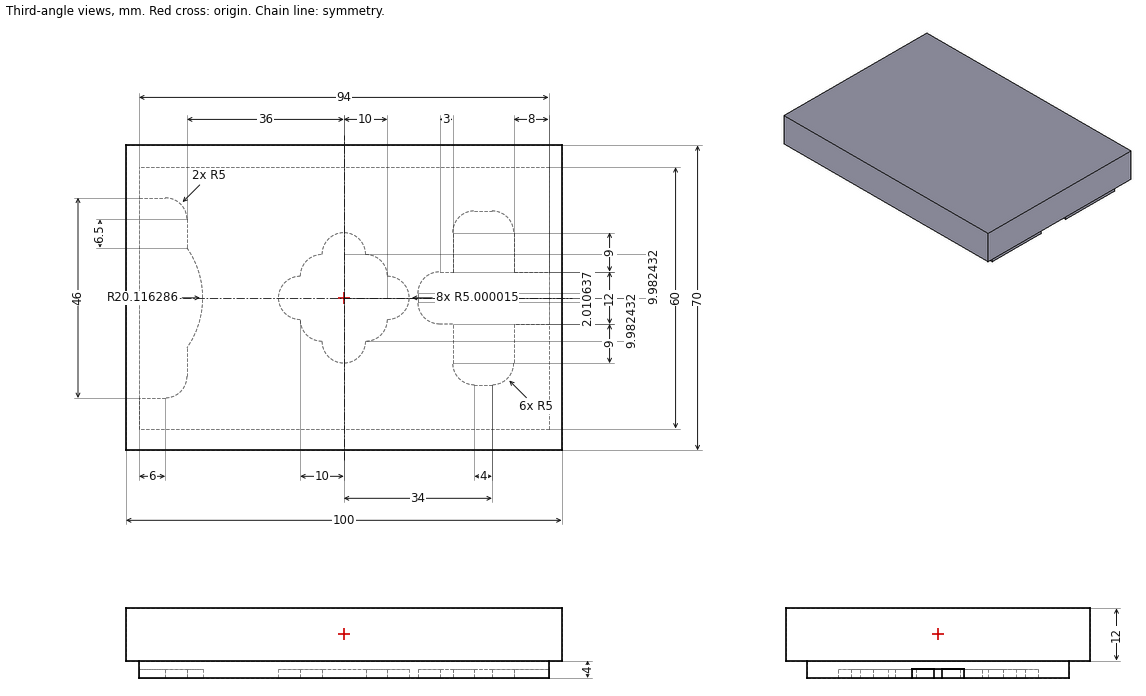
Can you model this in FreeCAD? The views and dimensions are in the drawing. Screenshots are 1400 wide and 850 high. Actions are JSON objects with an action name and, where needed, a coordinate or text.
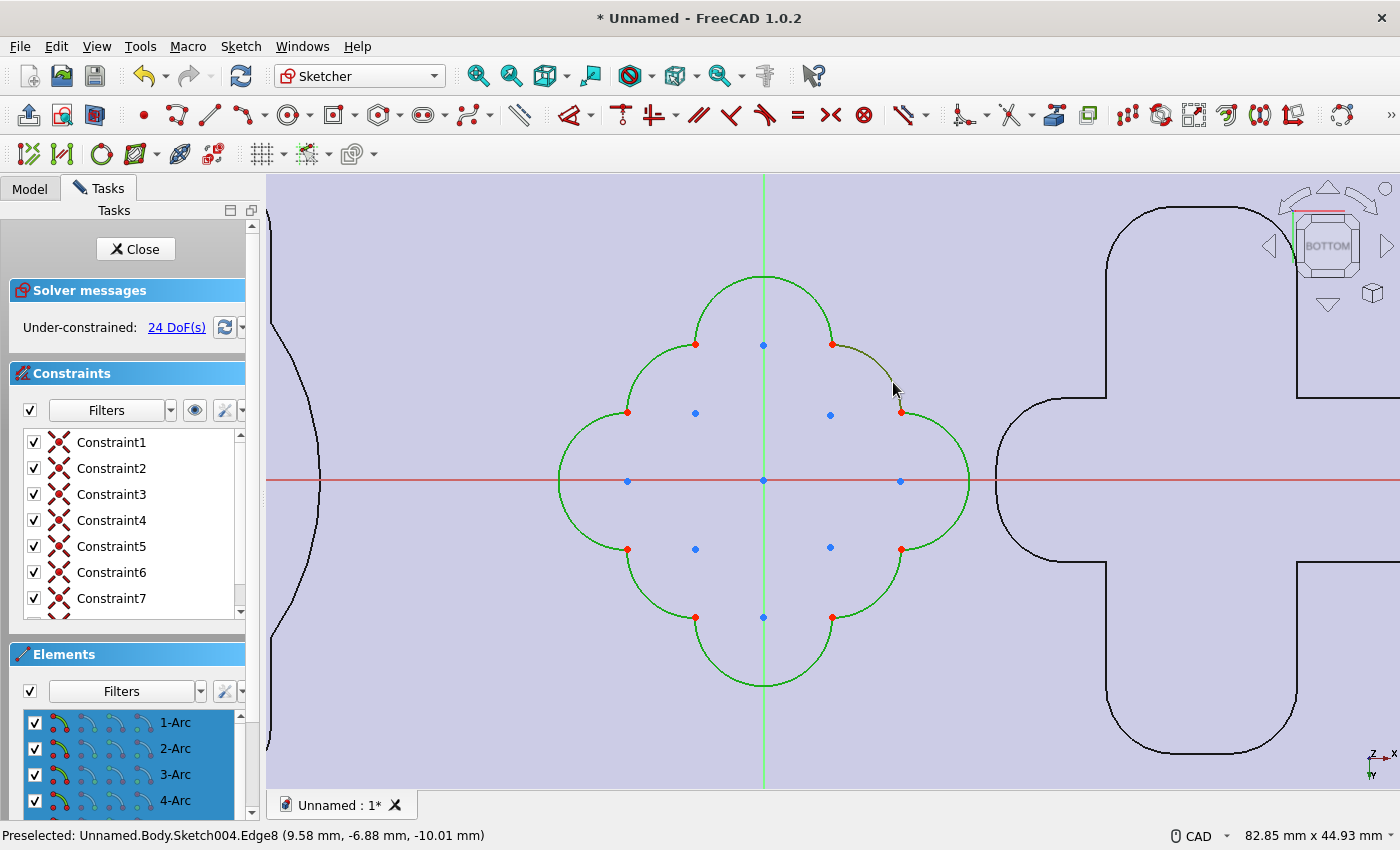
{"action": "left_click", "coordinate": [798, 116]}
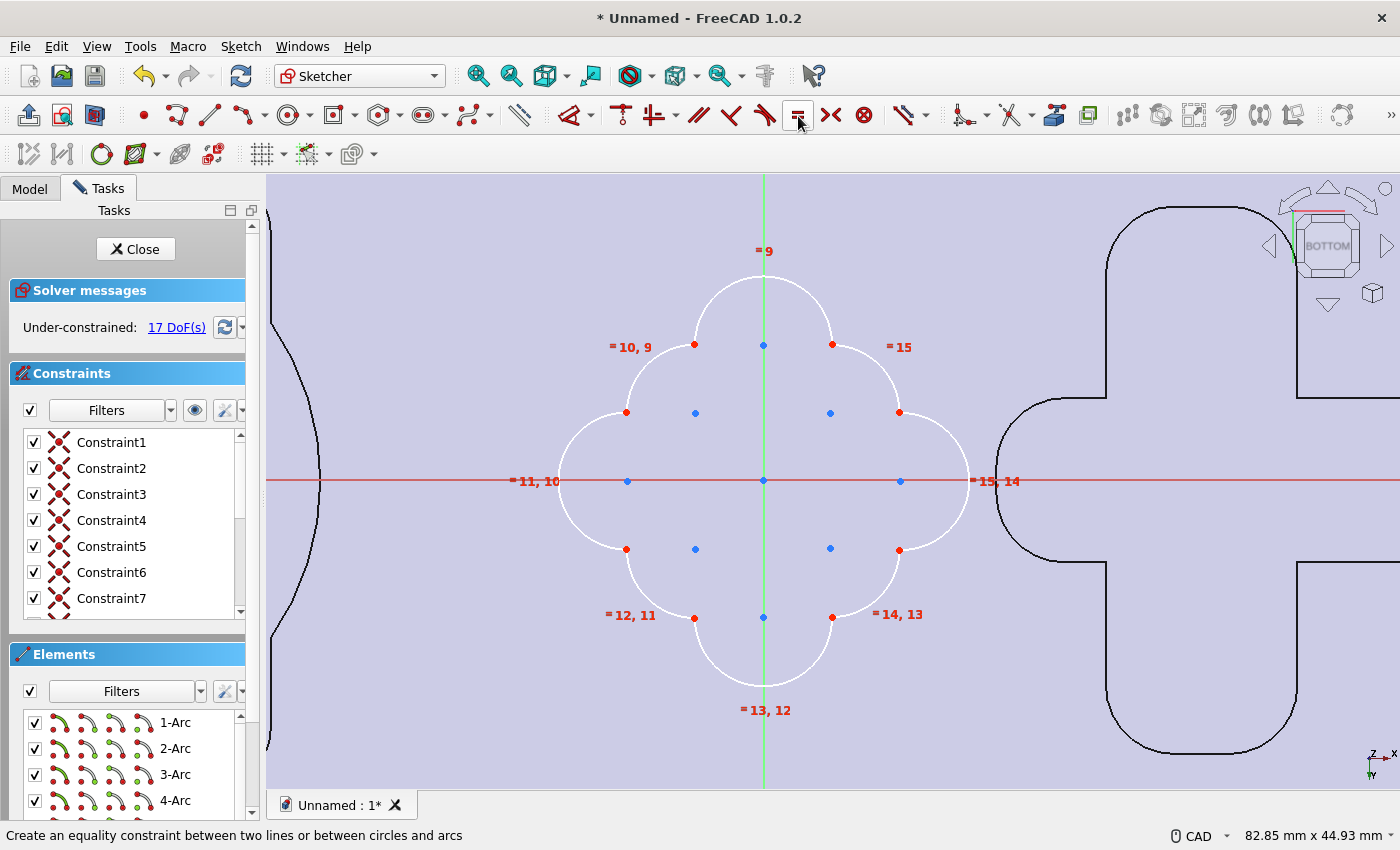
{"action": "left_click", "coordinate": [764, 345]}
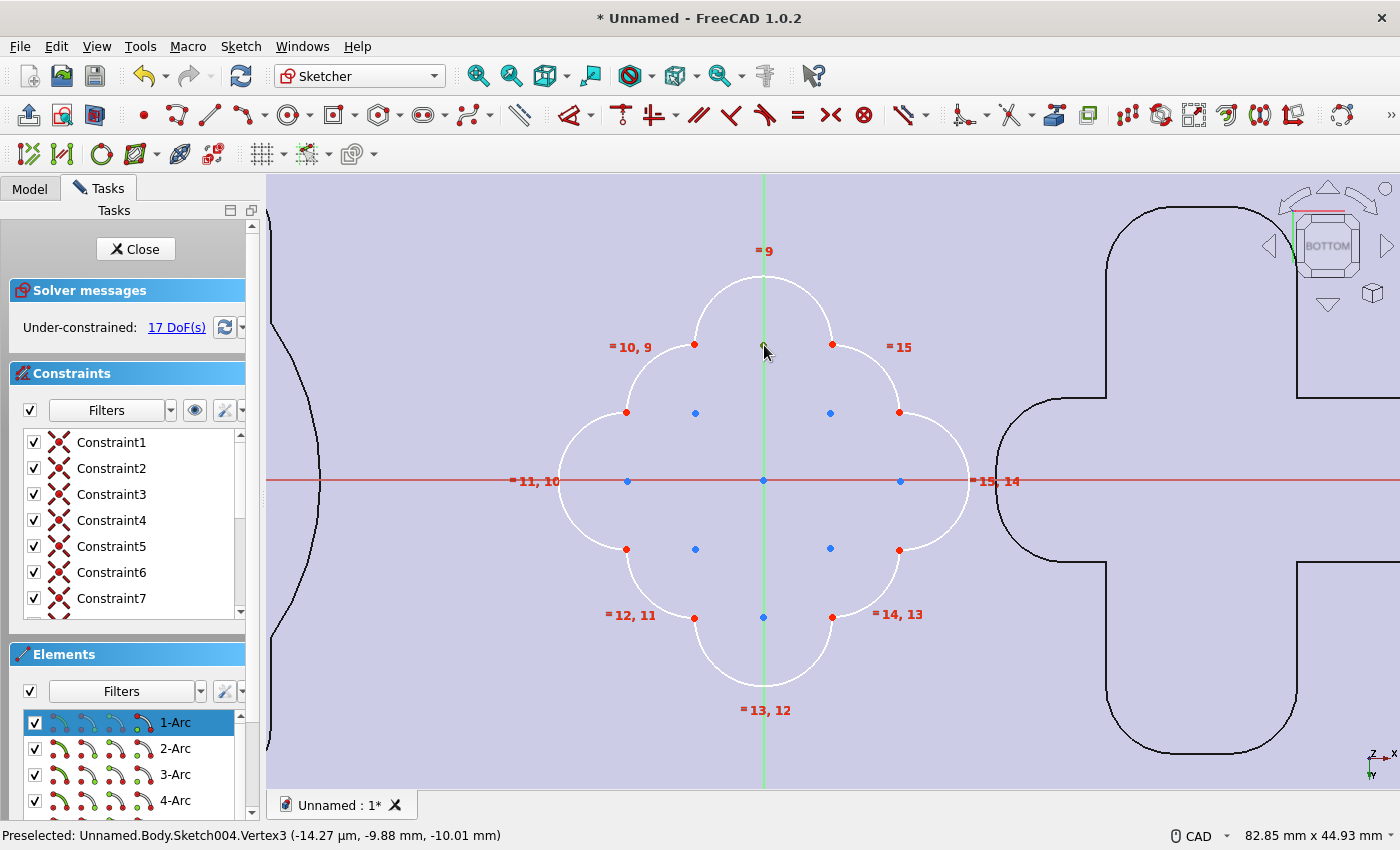
{"action": "left_click", "coordinate": [764, 721]}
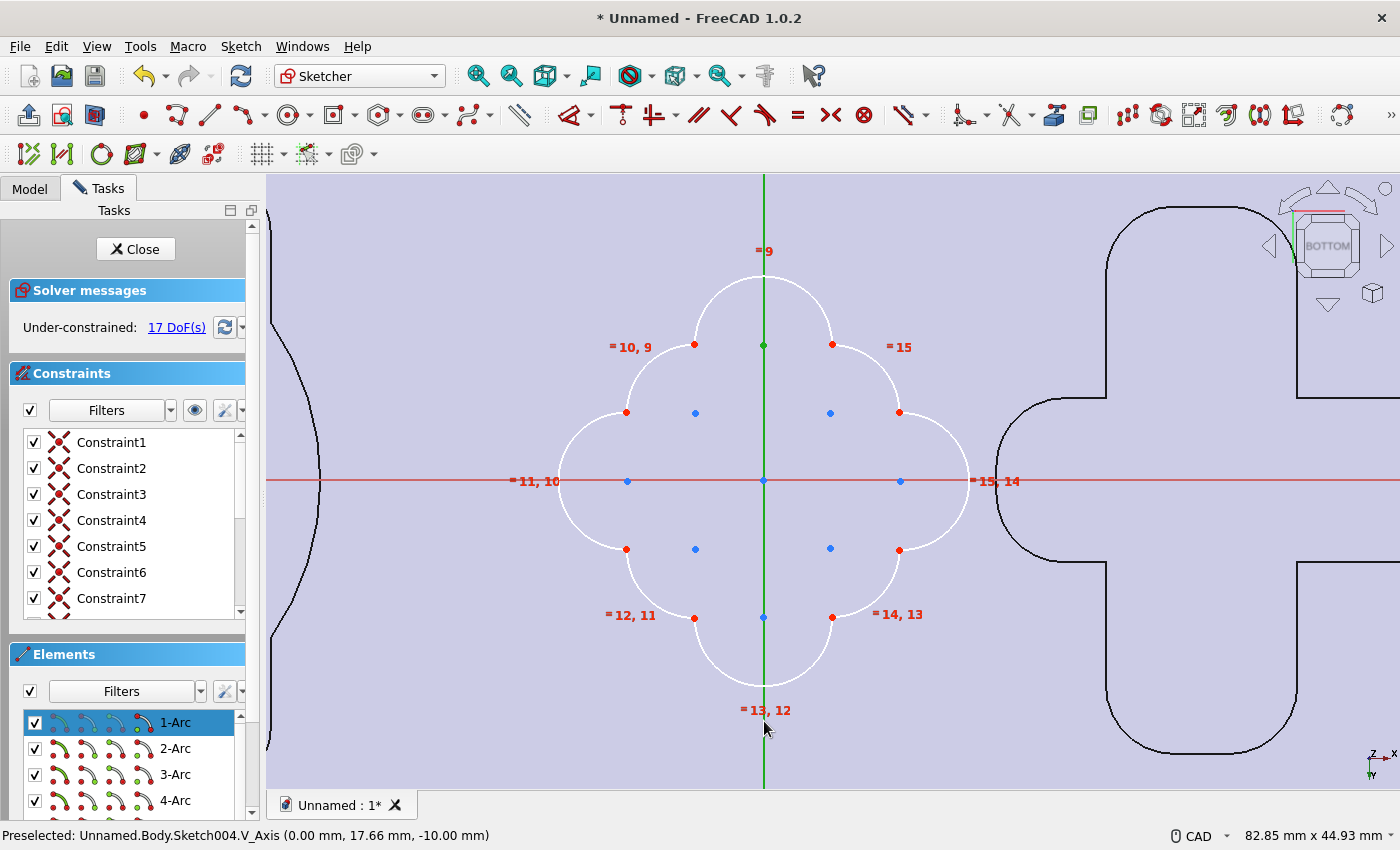
{"action": "left_click", "coordinate": [621, 116]}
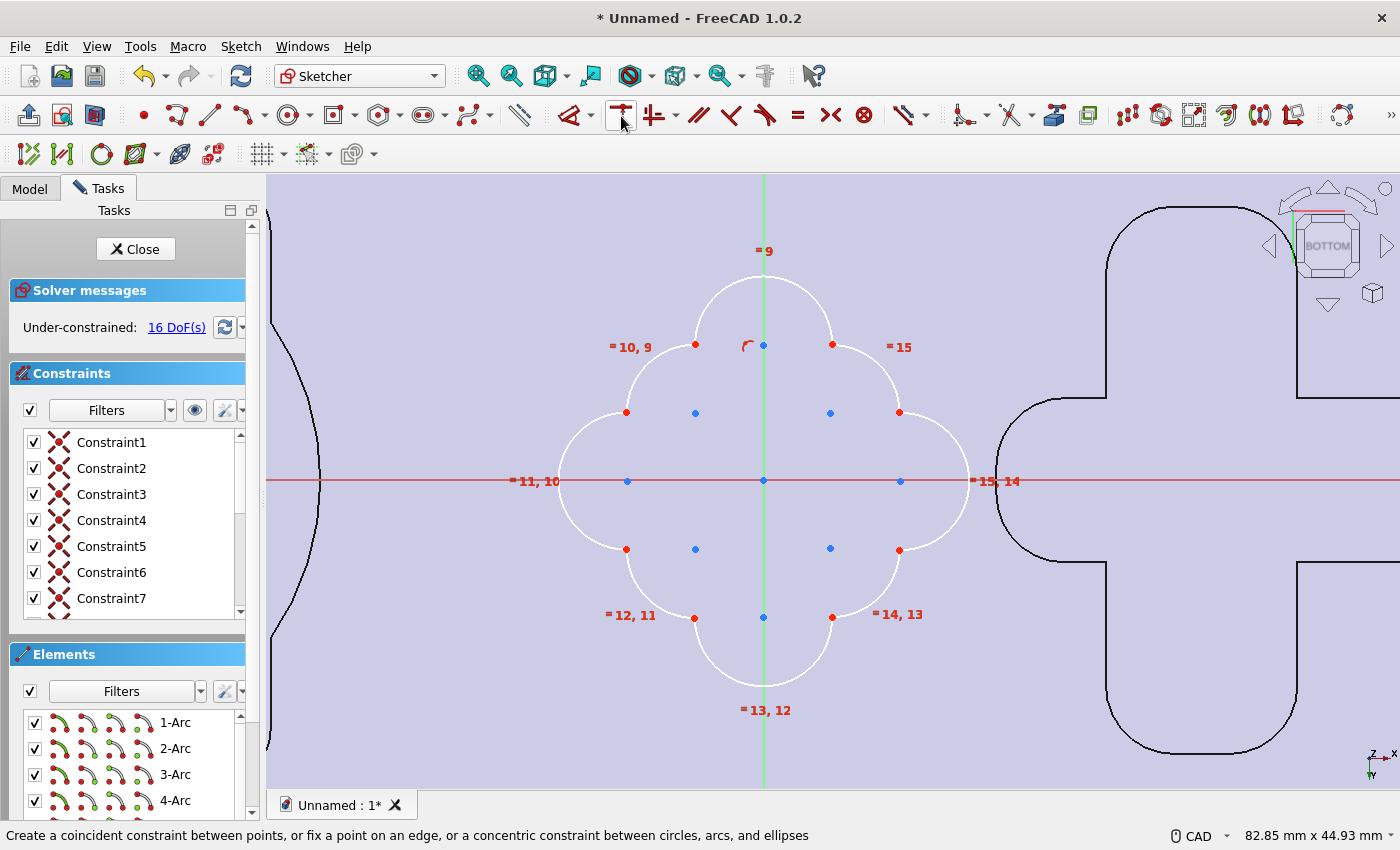
{"action": "left_click", "coordinate": [627, 481]}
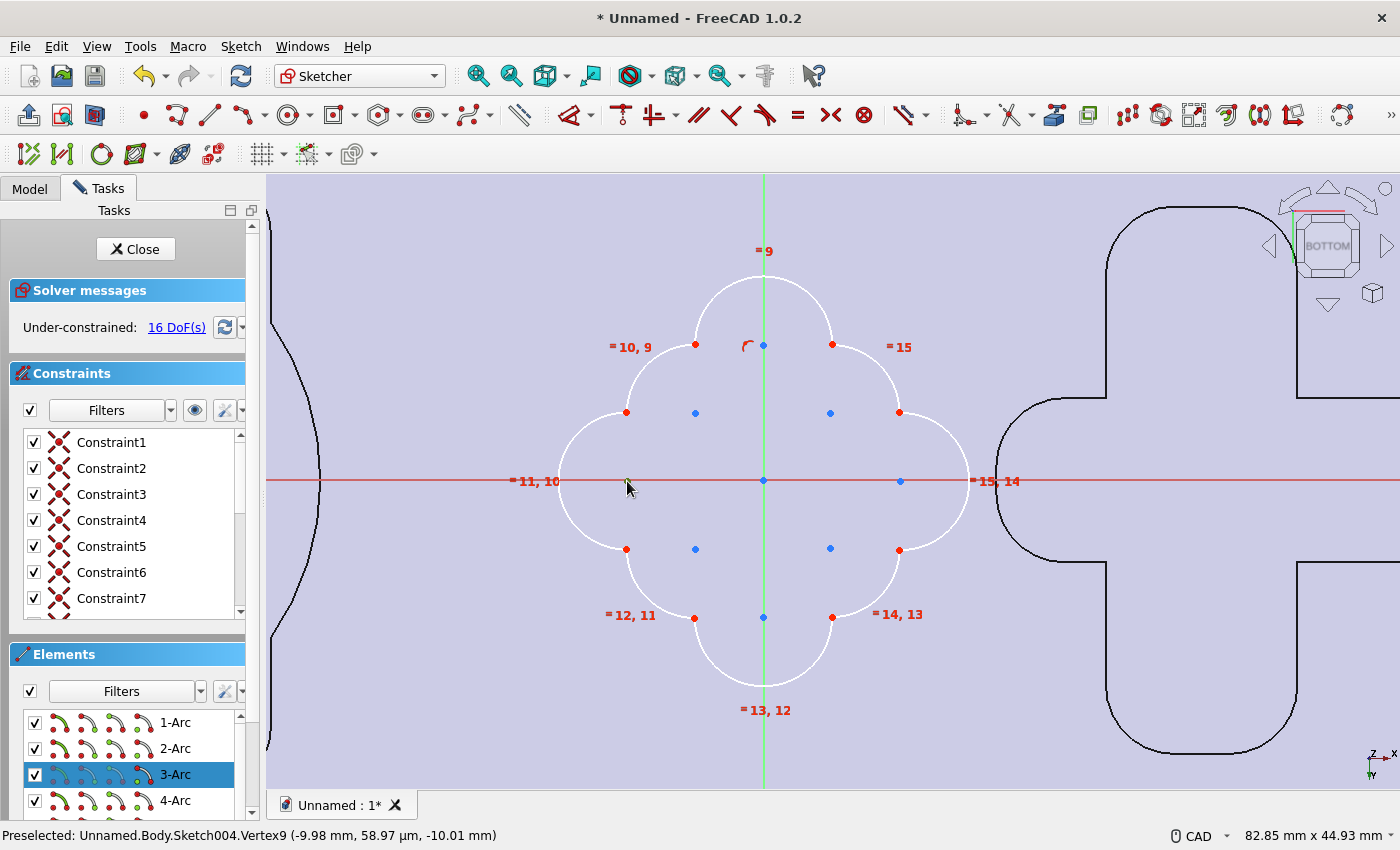
{"action": "left_click", "coordinate": [361, 480]}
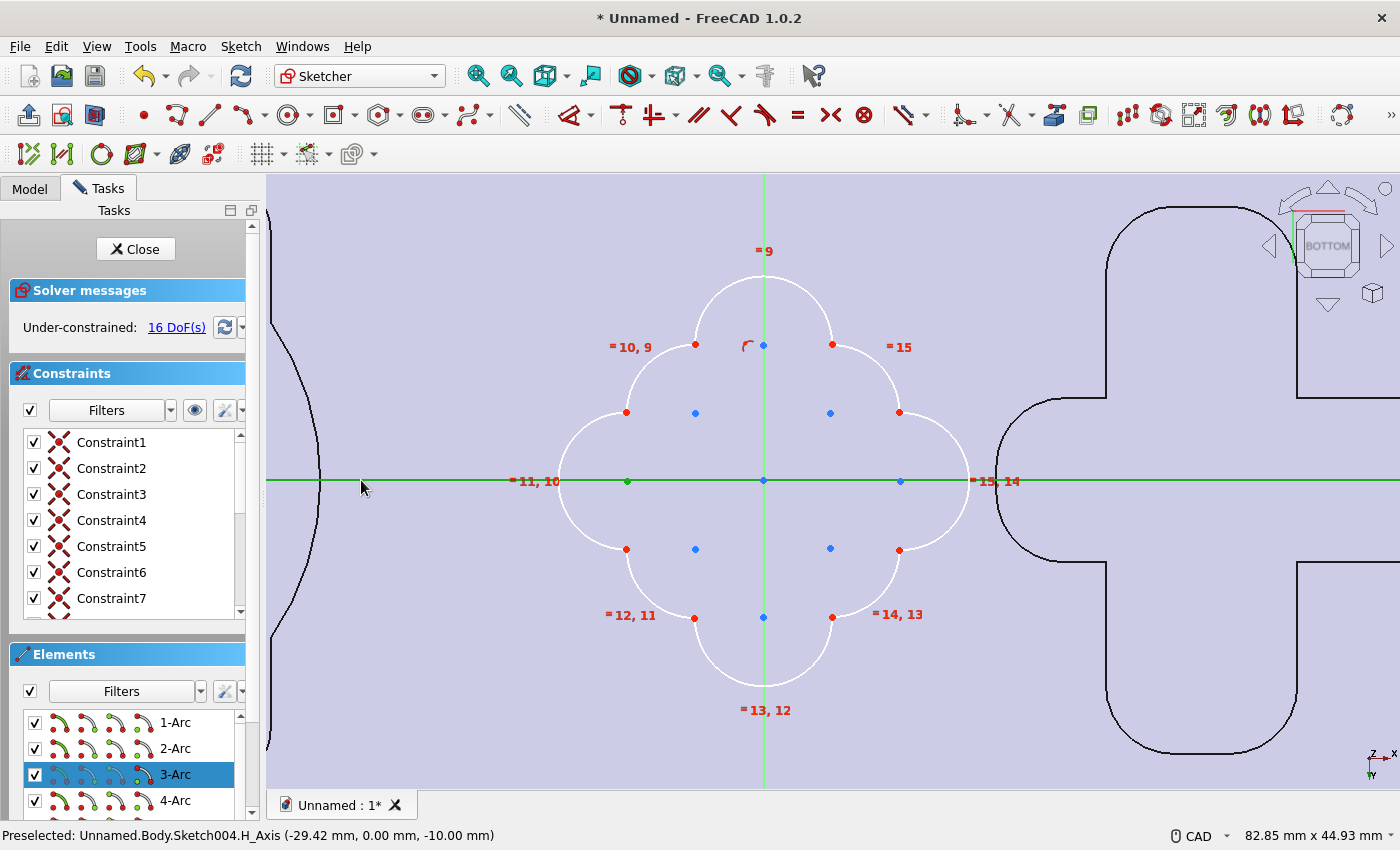
{"action": "left_click", "coordinate": [621, 116]}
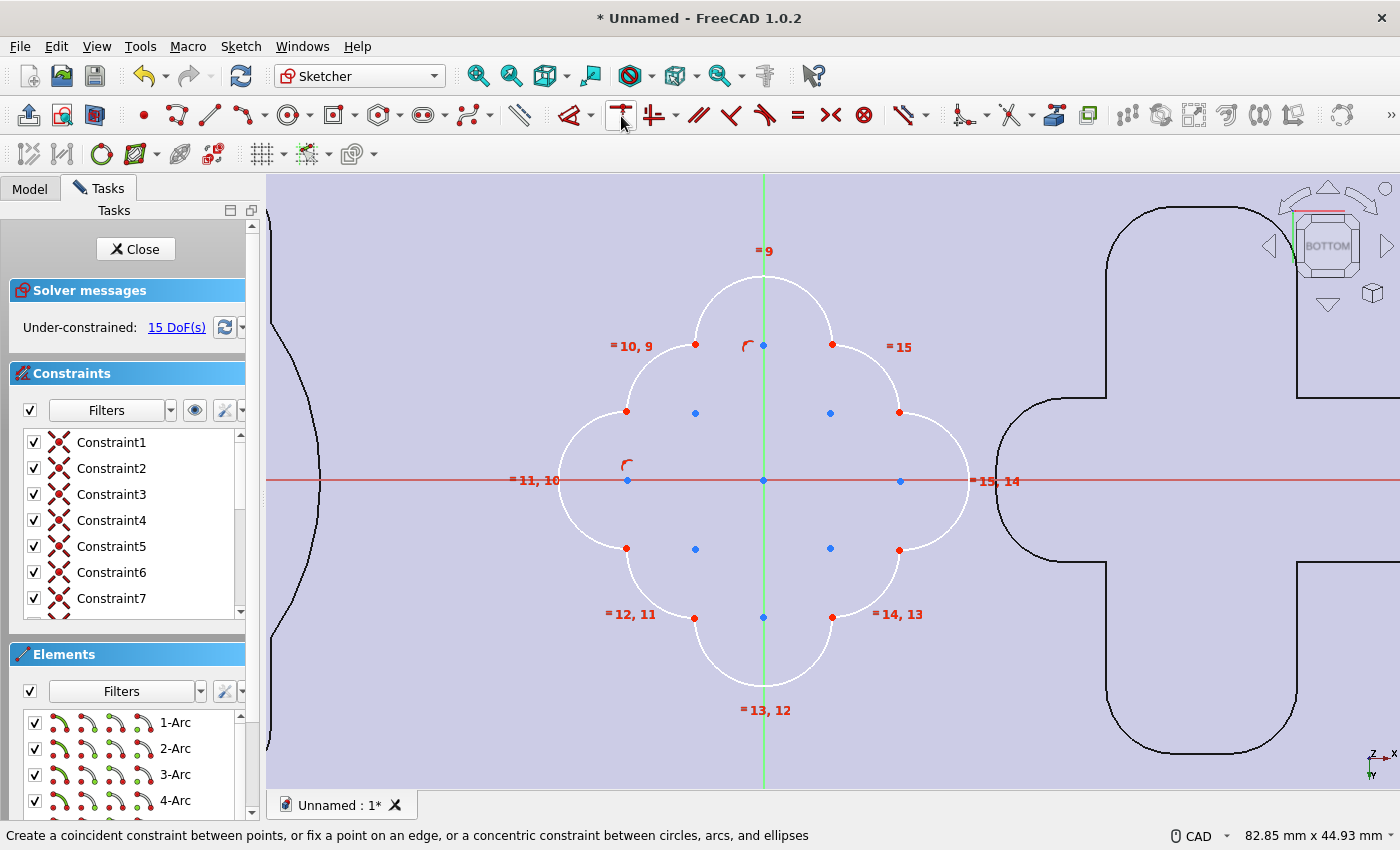
{"action": "left_click", "coordinate": [764, 618]}